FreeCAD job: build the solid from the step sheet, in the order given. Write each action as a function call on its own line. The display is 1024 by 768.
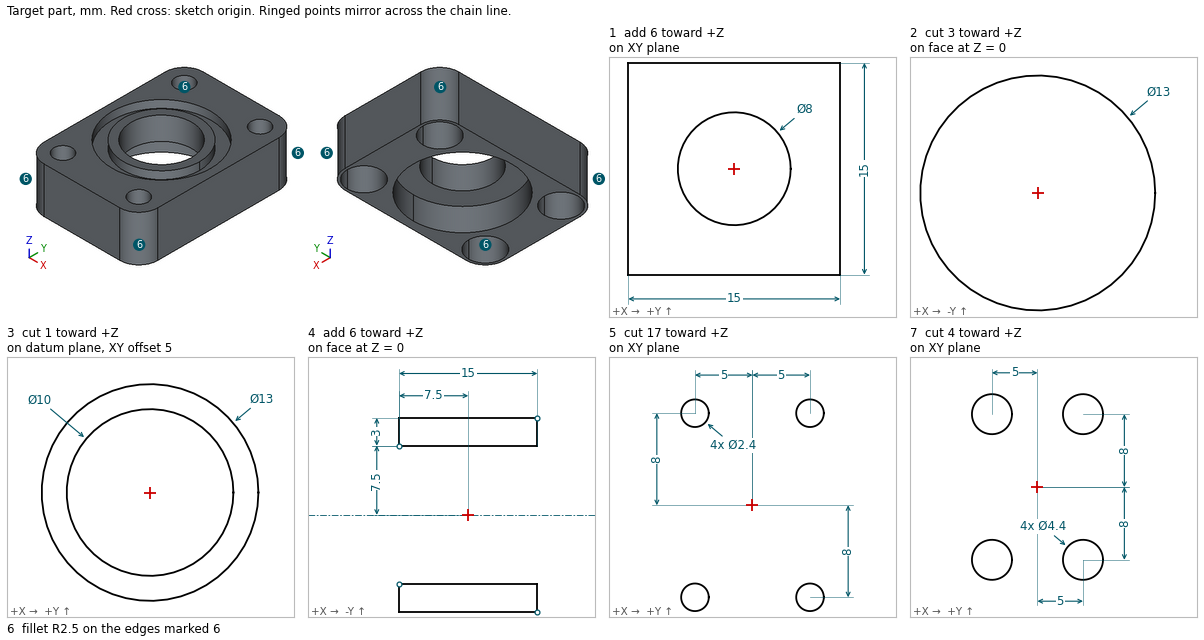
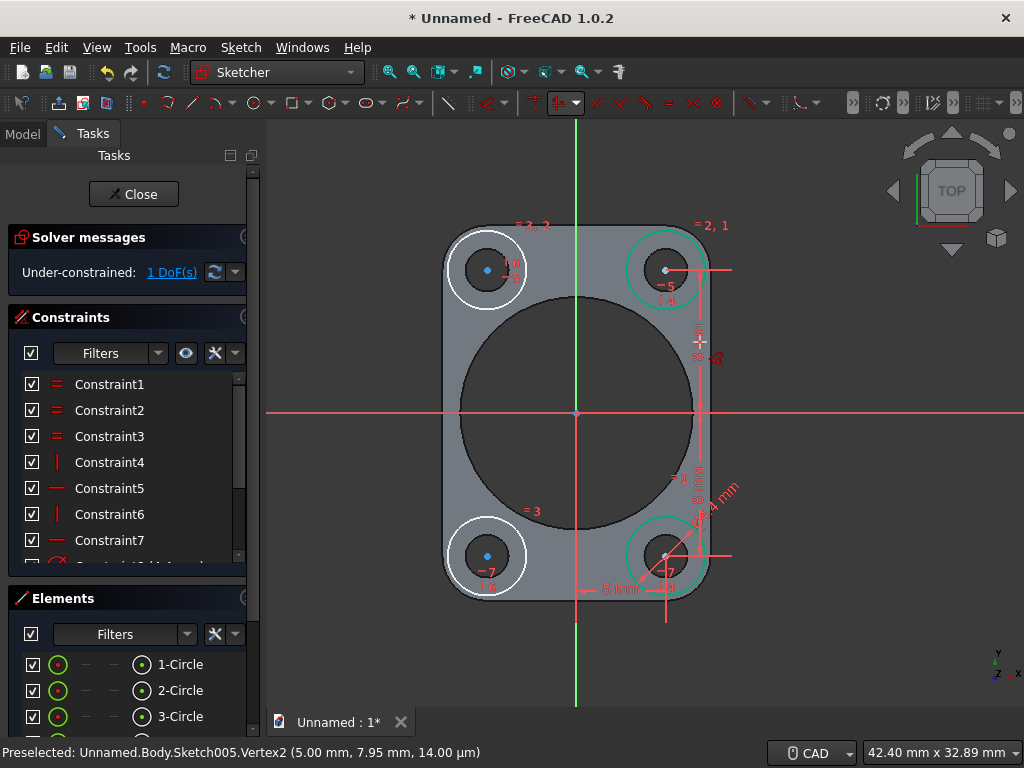
click(487, 270)
click(532, 236)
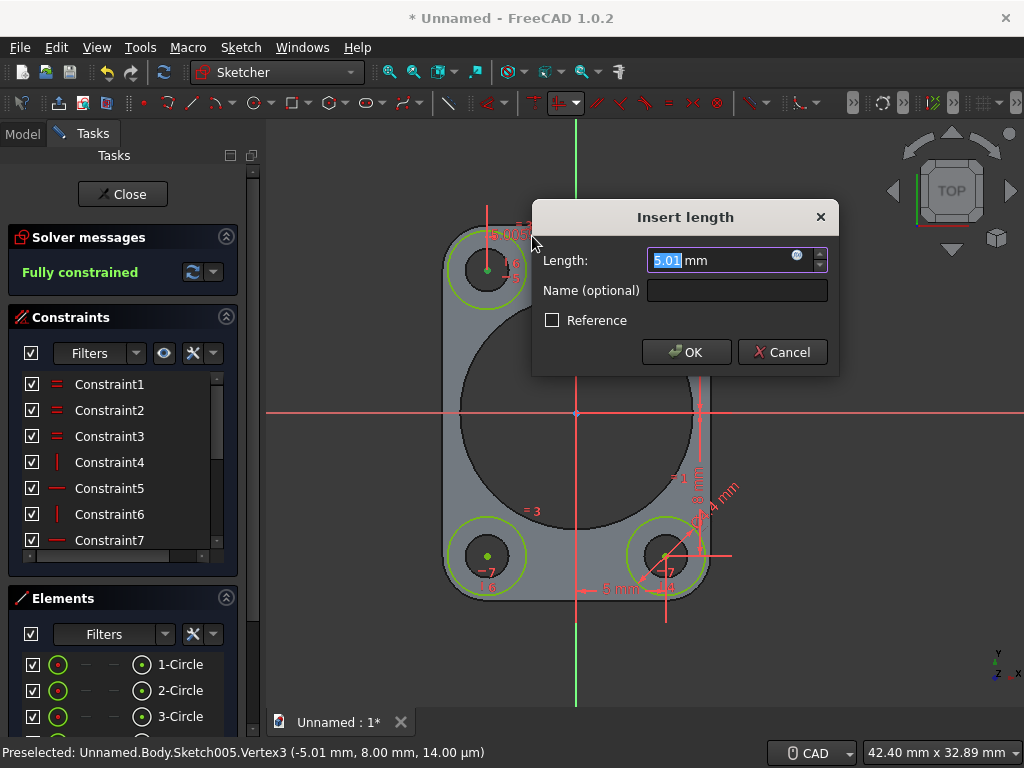
text(5)
key(Return)
key(Escape)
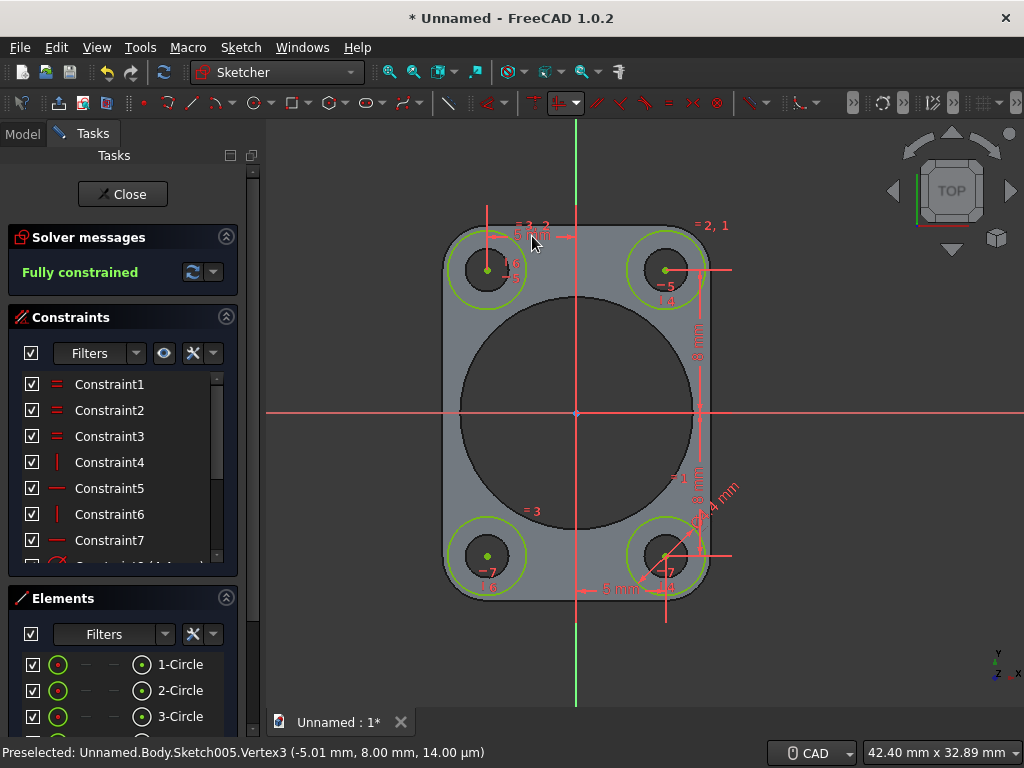
click(123, 194)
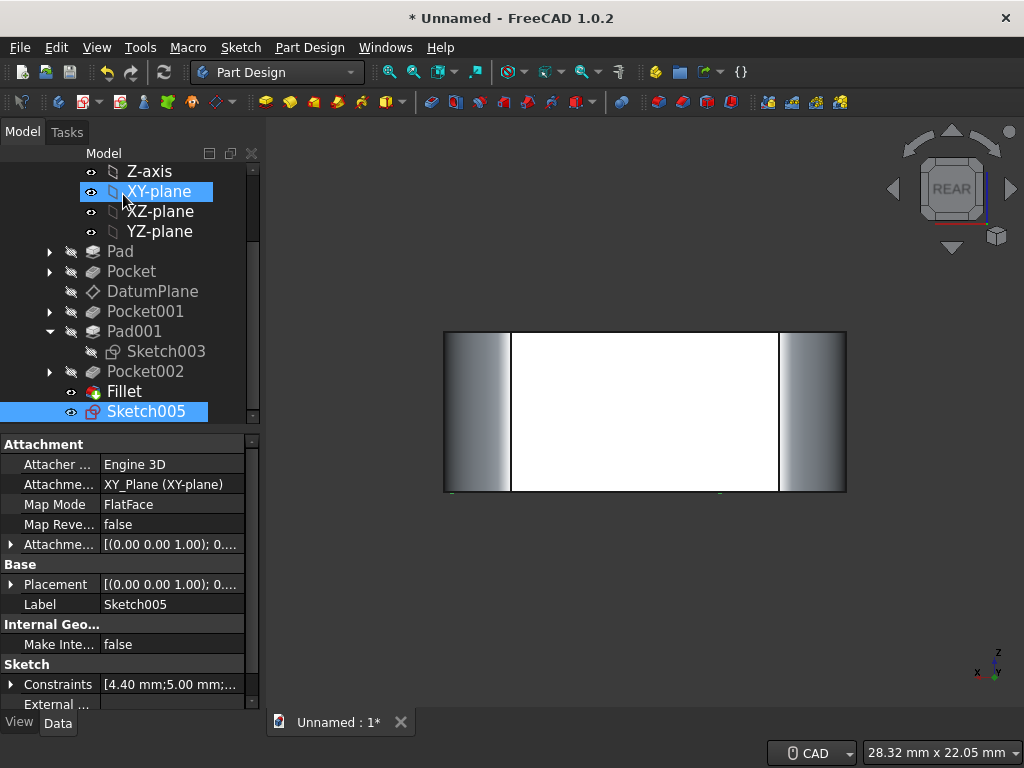
click(432, 102)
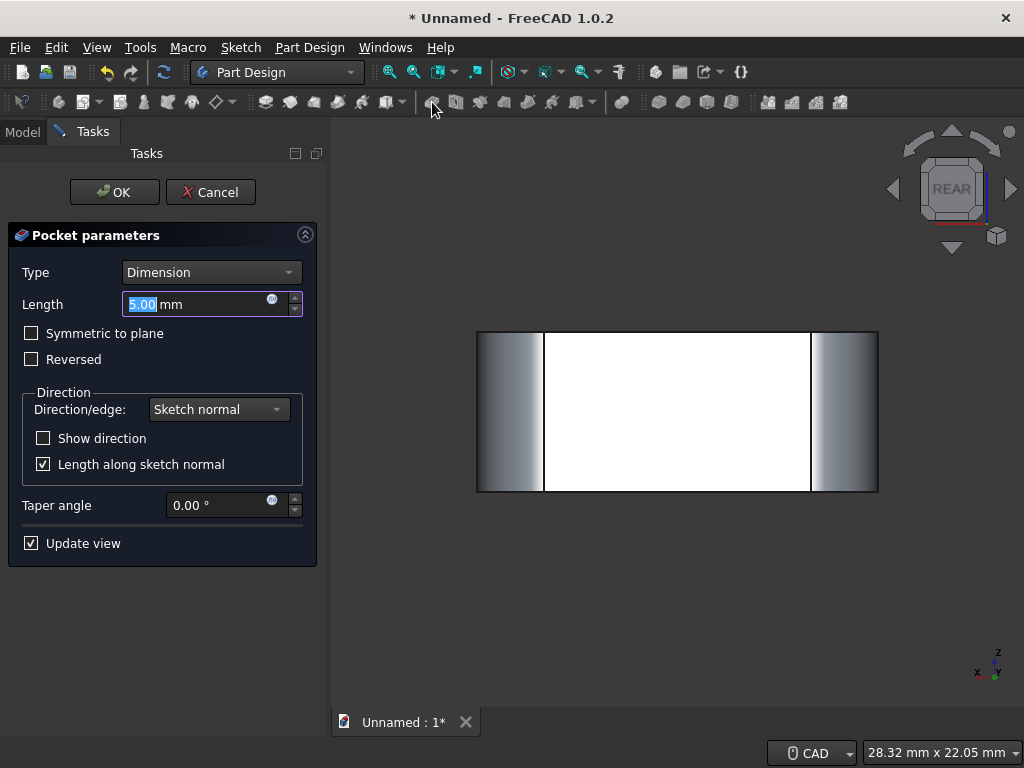
text(4)
key(Tab)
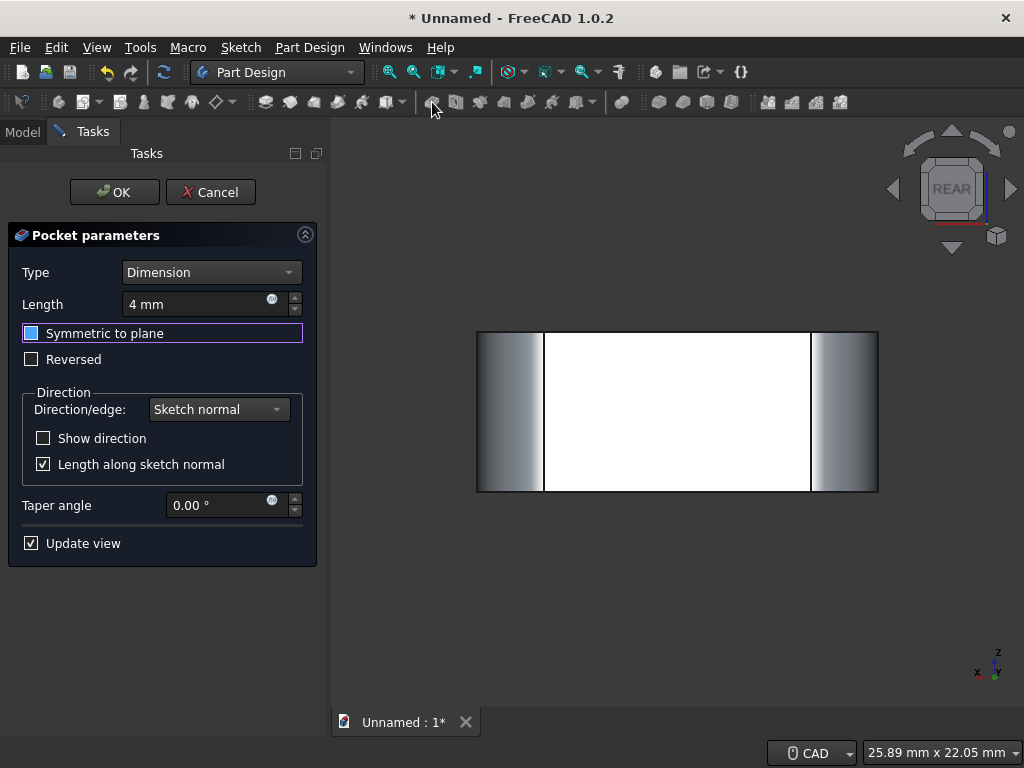
click(30, 359)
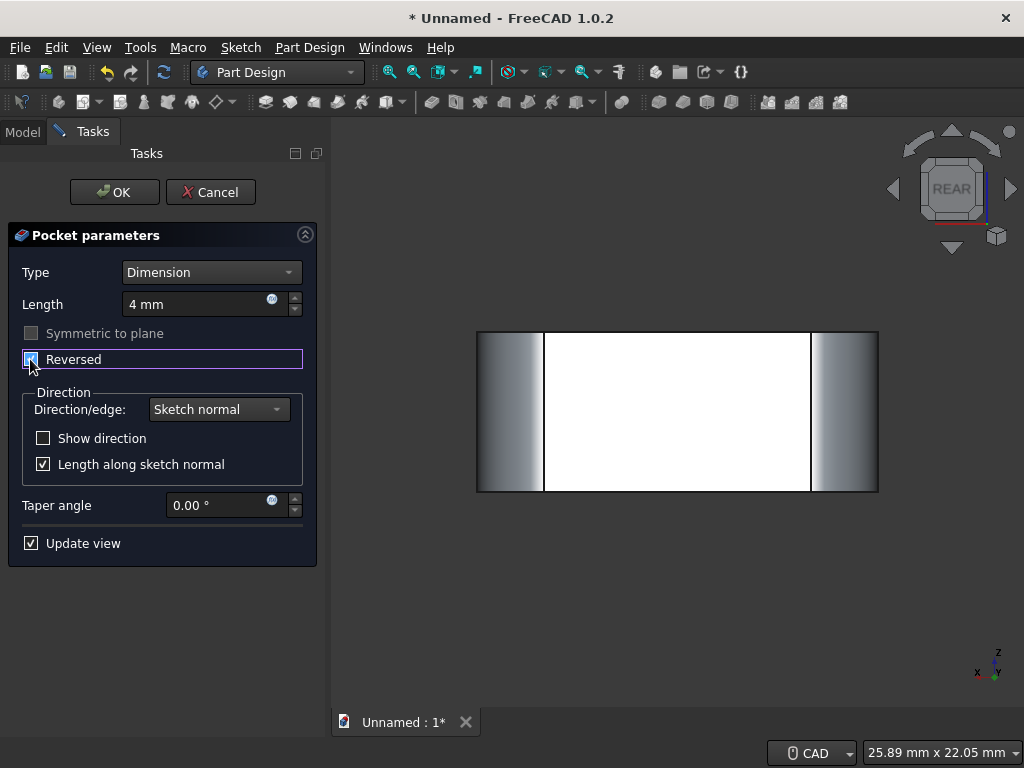
click(115, 192)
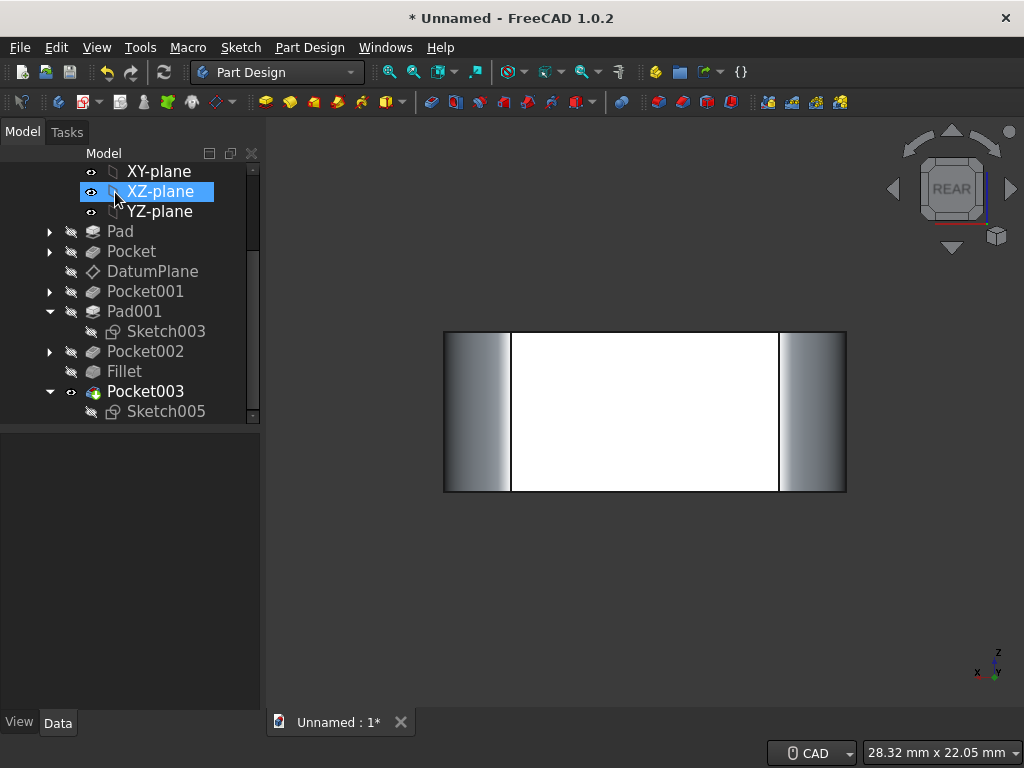
key(0)